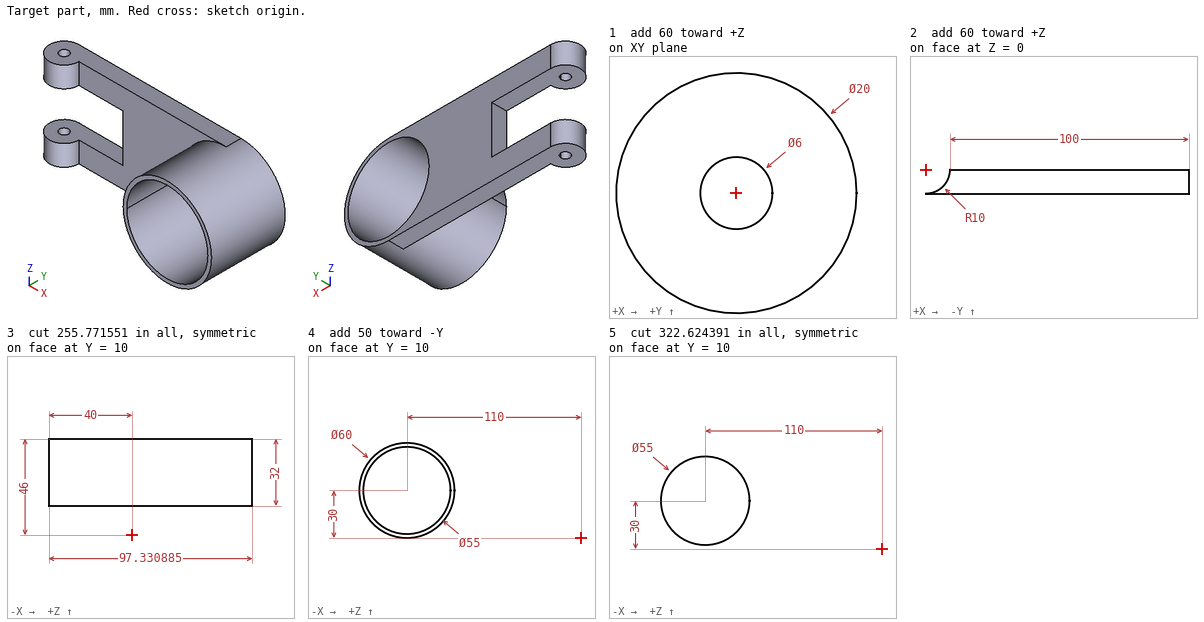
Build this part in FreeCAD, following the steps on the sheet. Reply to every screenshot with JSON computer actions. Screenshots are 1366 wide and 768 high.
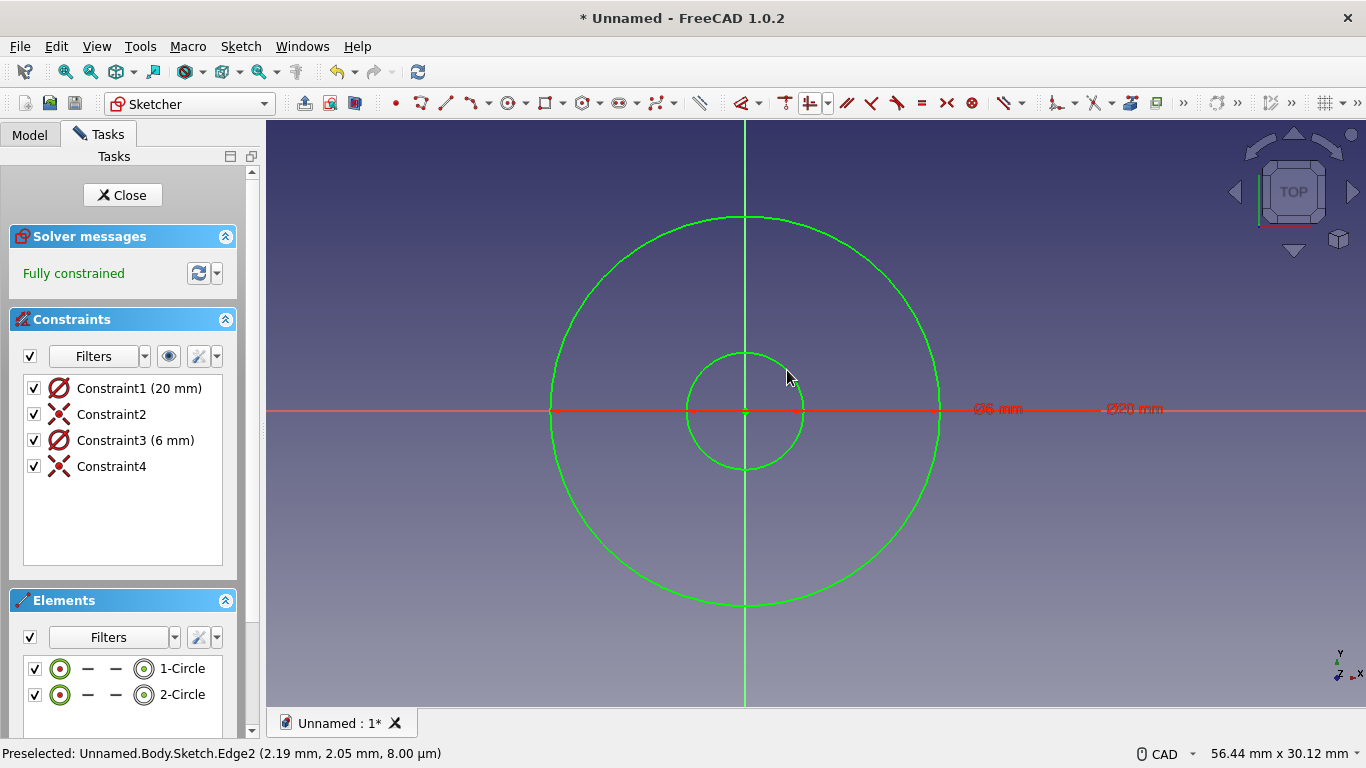
{"action": "left_click", "coordinate": [123, 195]}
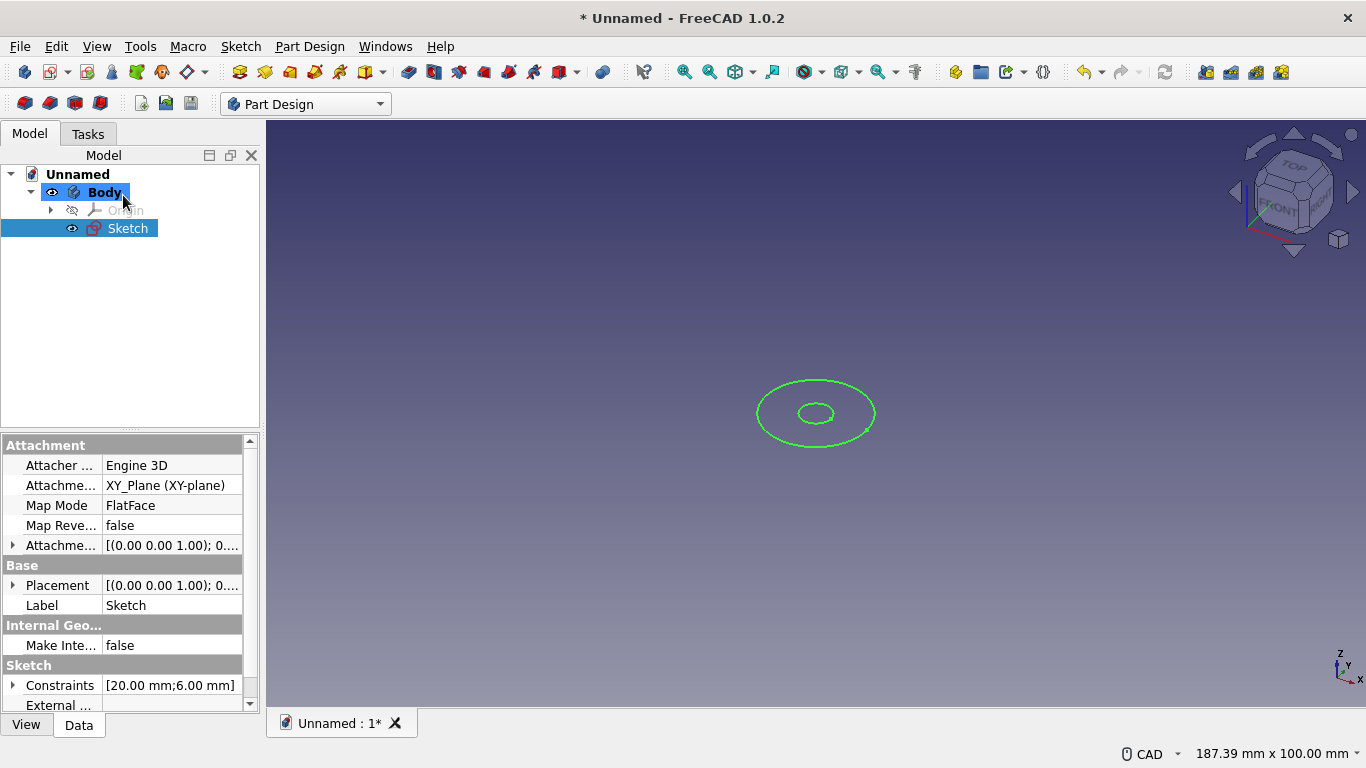
{"action": "left_click", "coordinate": [240, 72]}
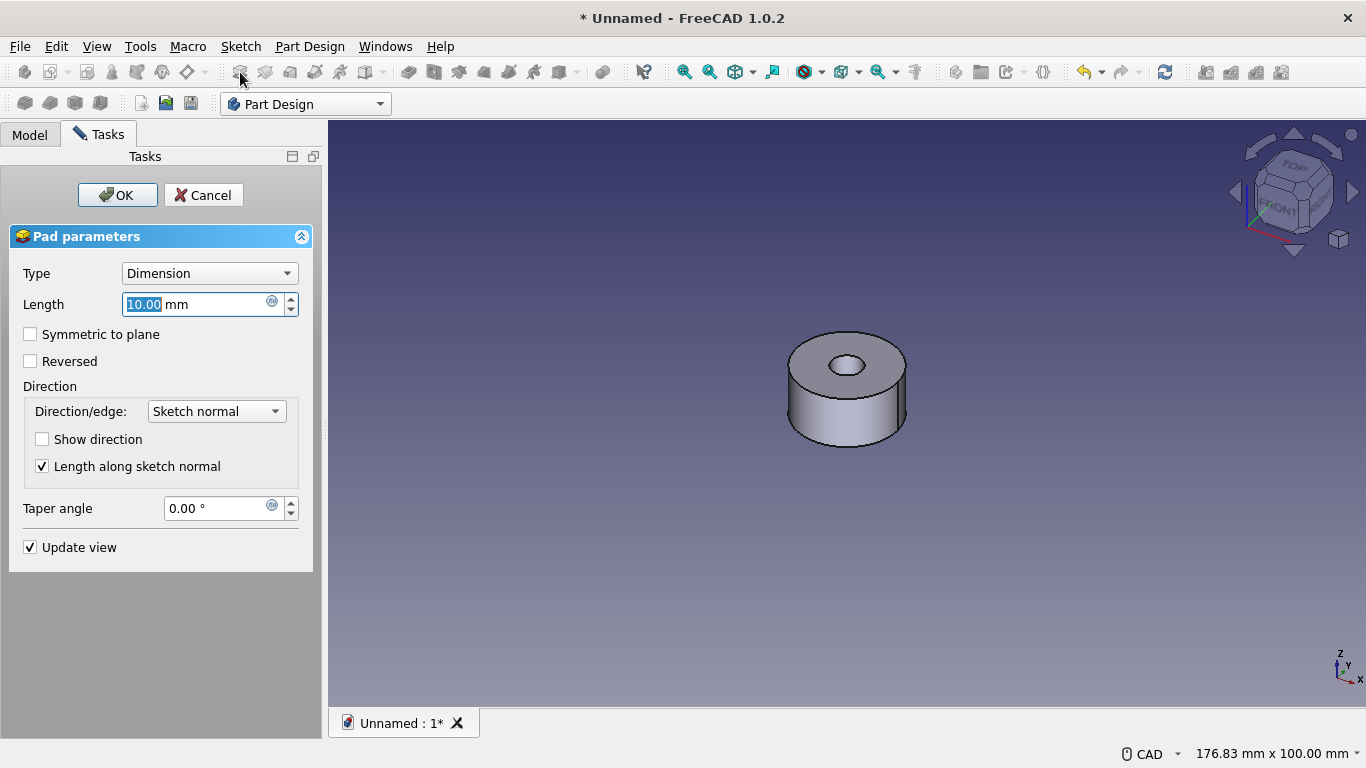
{"action": "type", "text": "60"}
{"action": "key", "text": "Tab"}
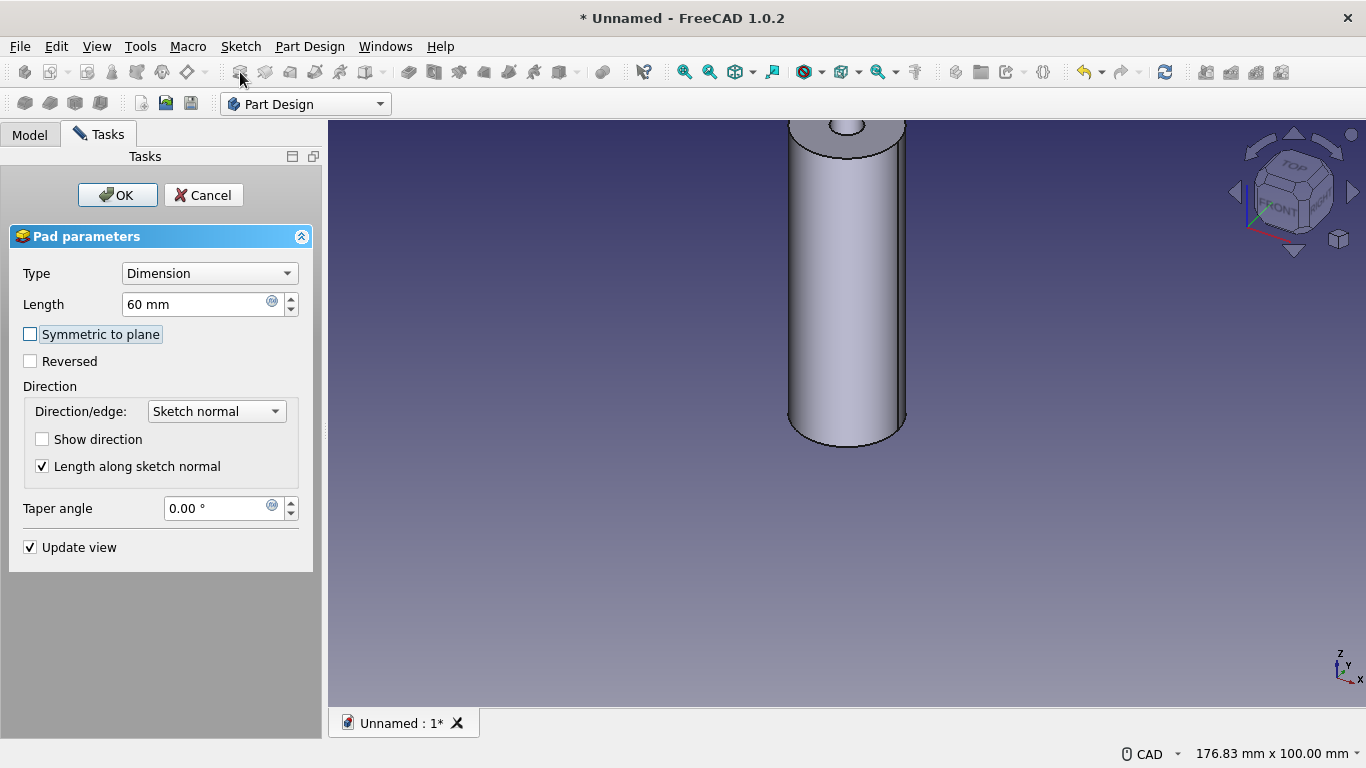
{"action": "left_click", "coordinate": [118, 195]}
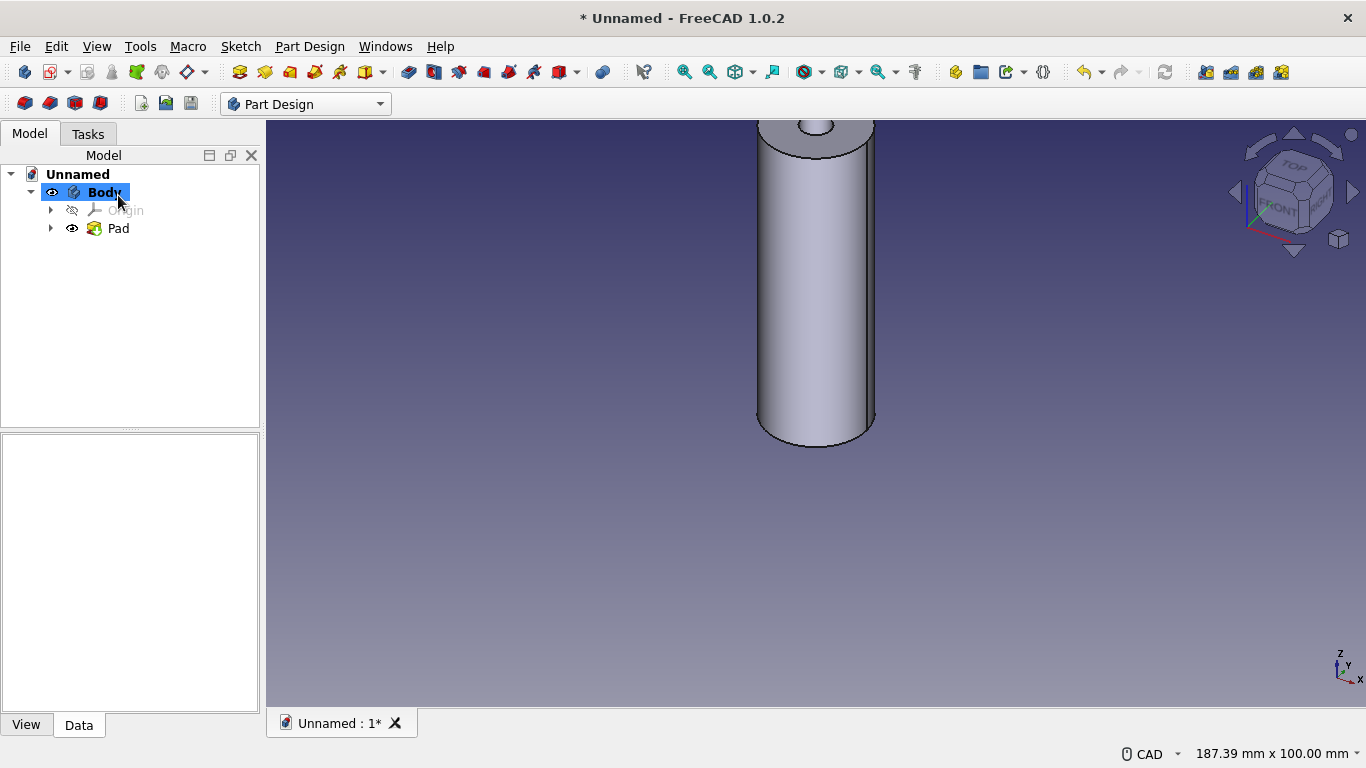
{"action": "left_click", "coordinate": [685, 72]}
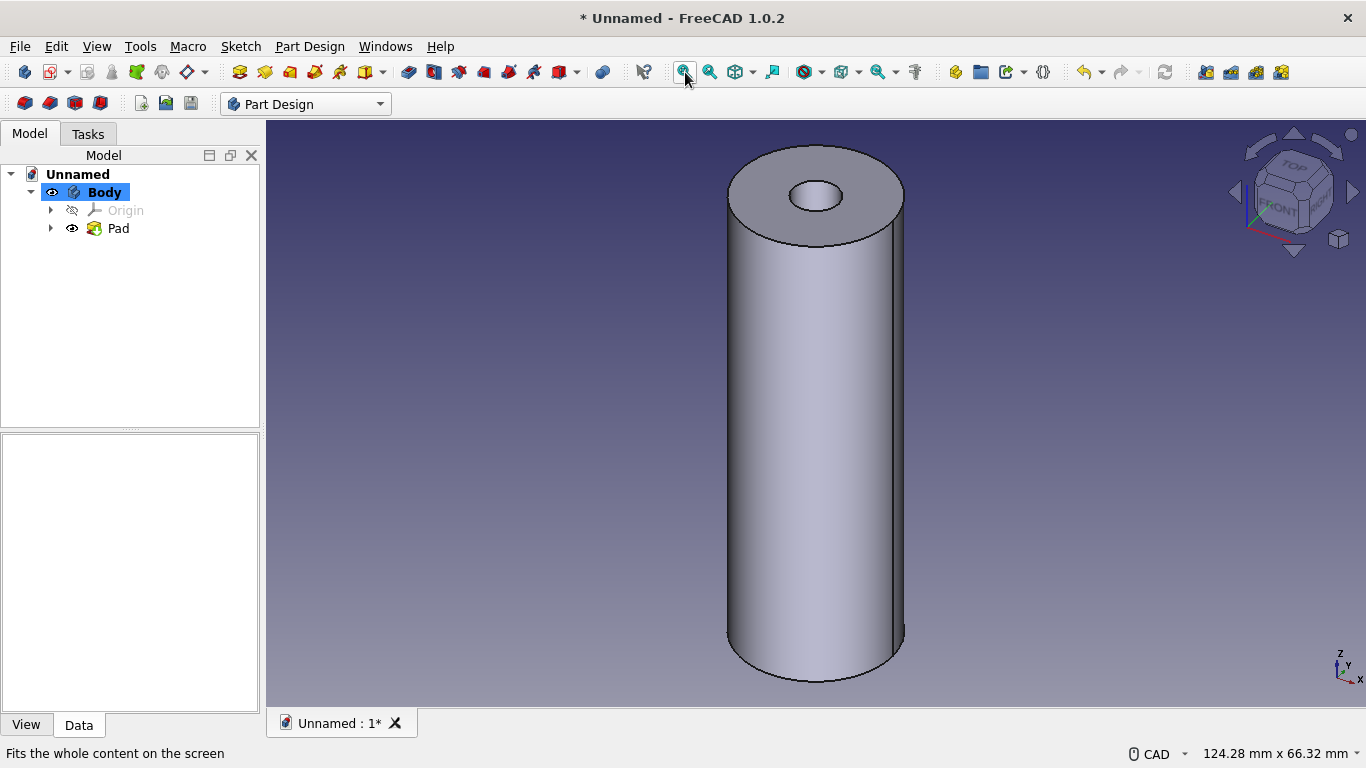
{"action": "key", "text": "5"}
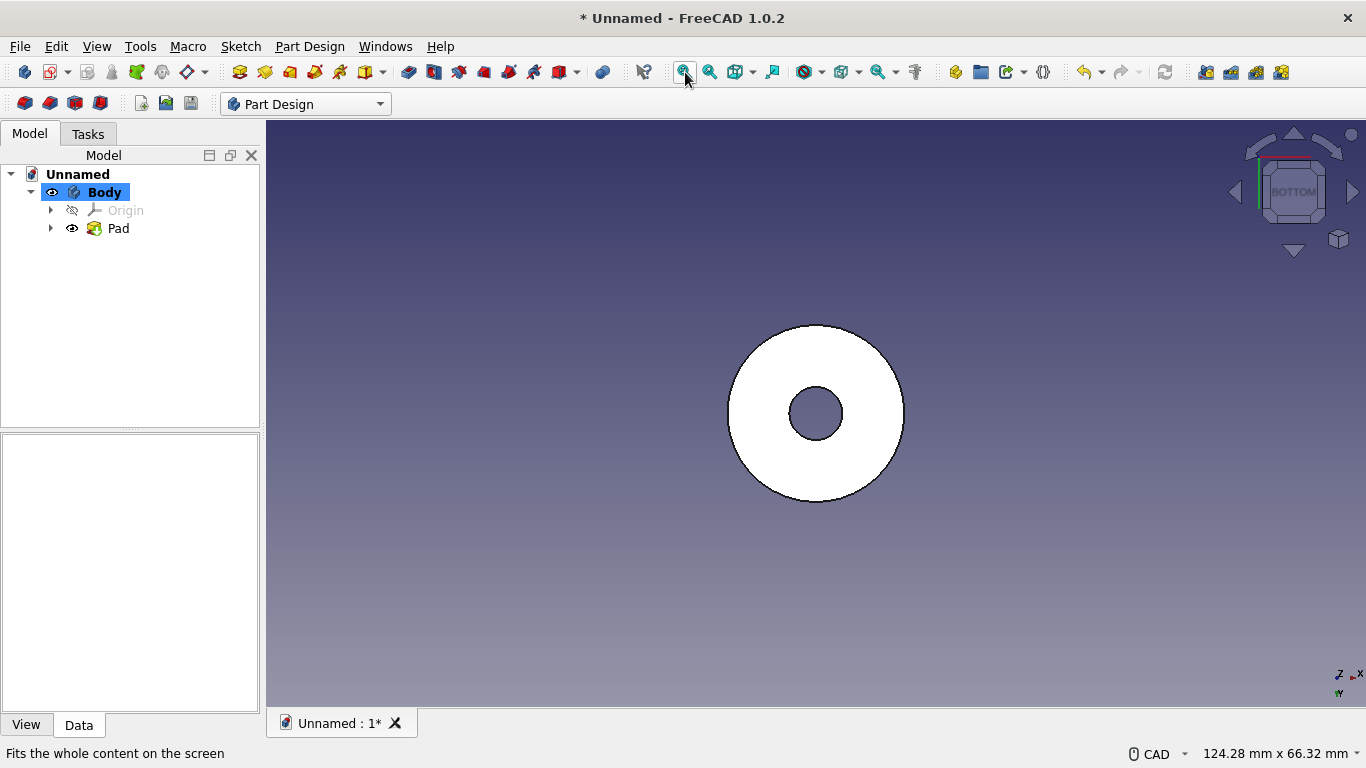
{"action": "left_click", "coordinate": [685, 72]}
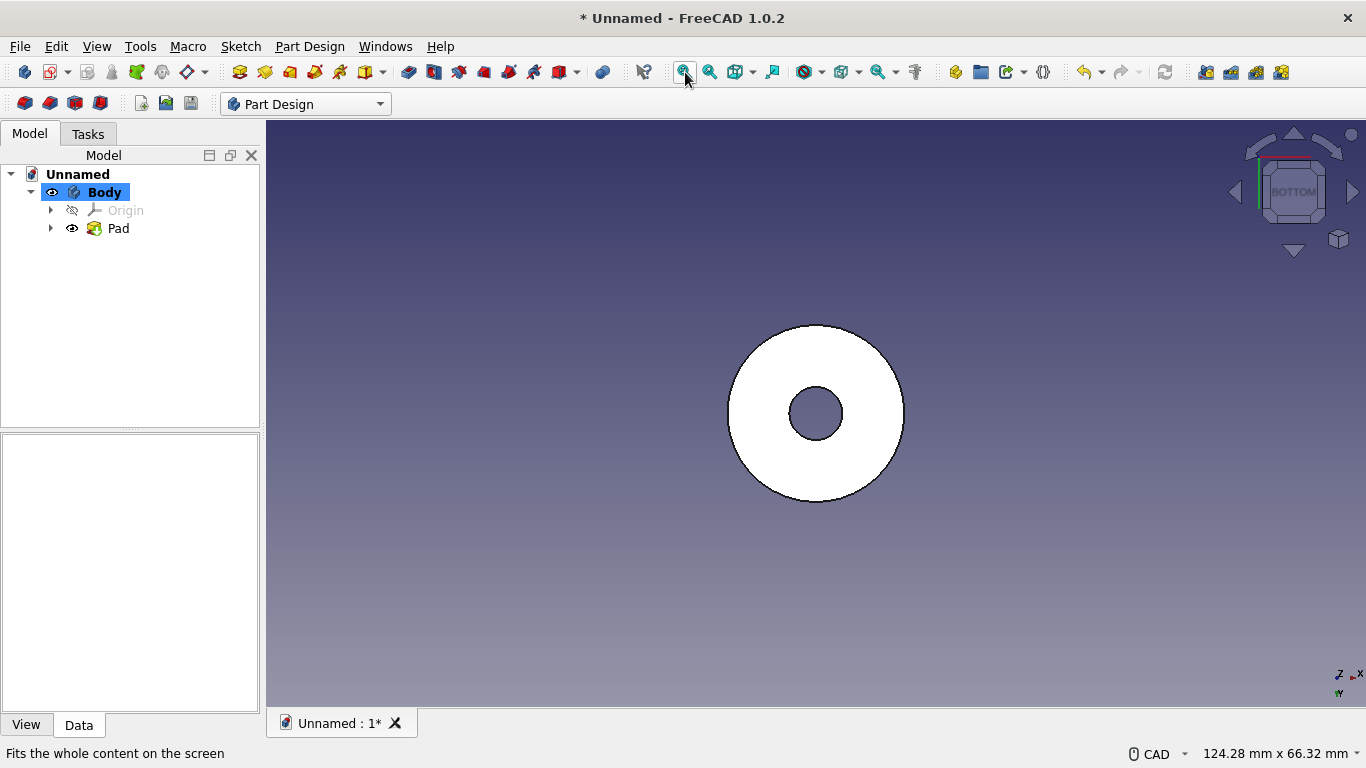
{"action": "left_click", "coordinate": [765, 438]}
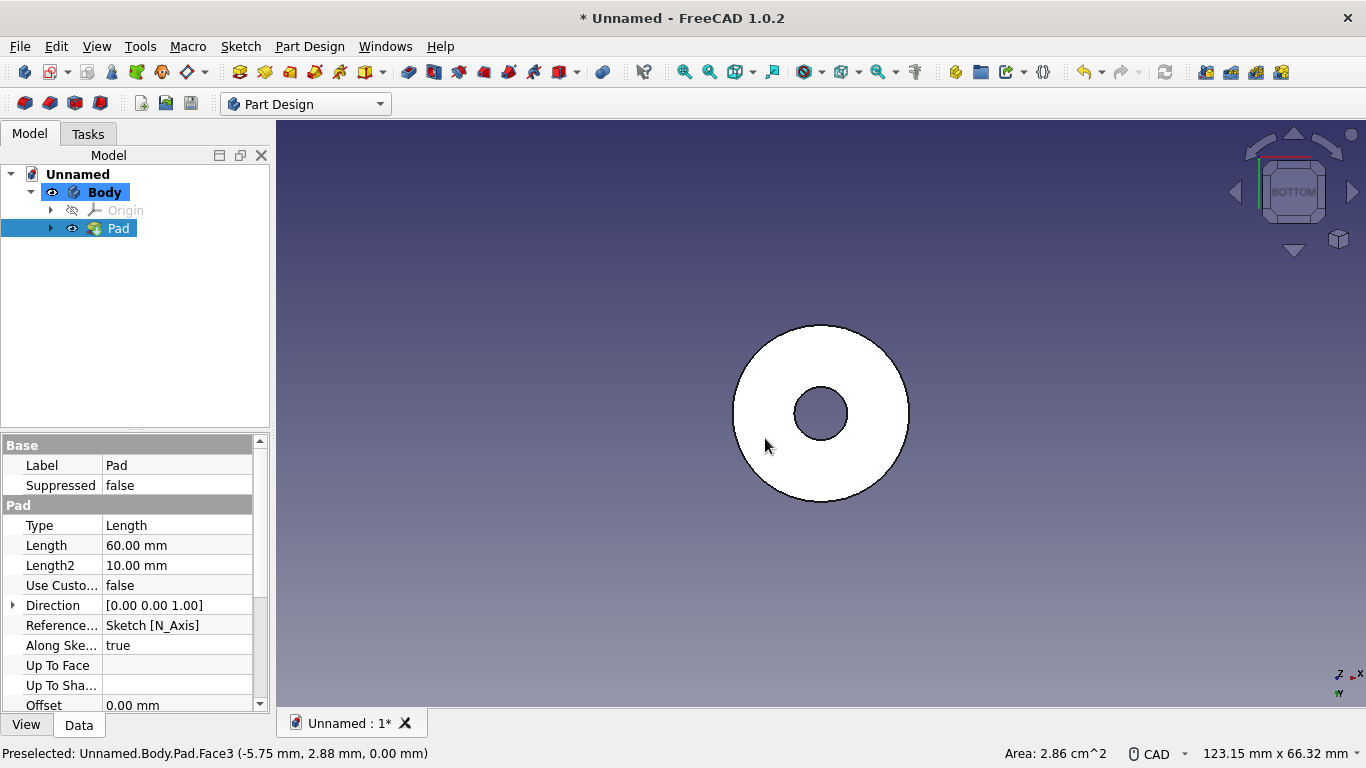
{"action": "left_click", "coordinate": [50, 72]}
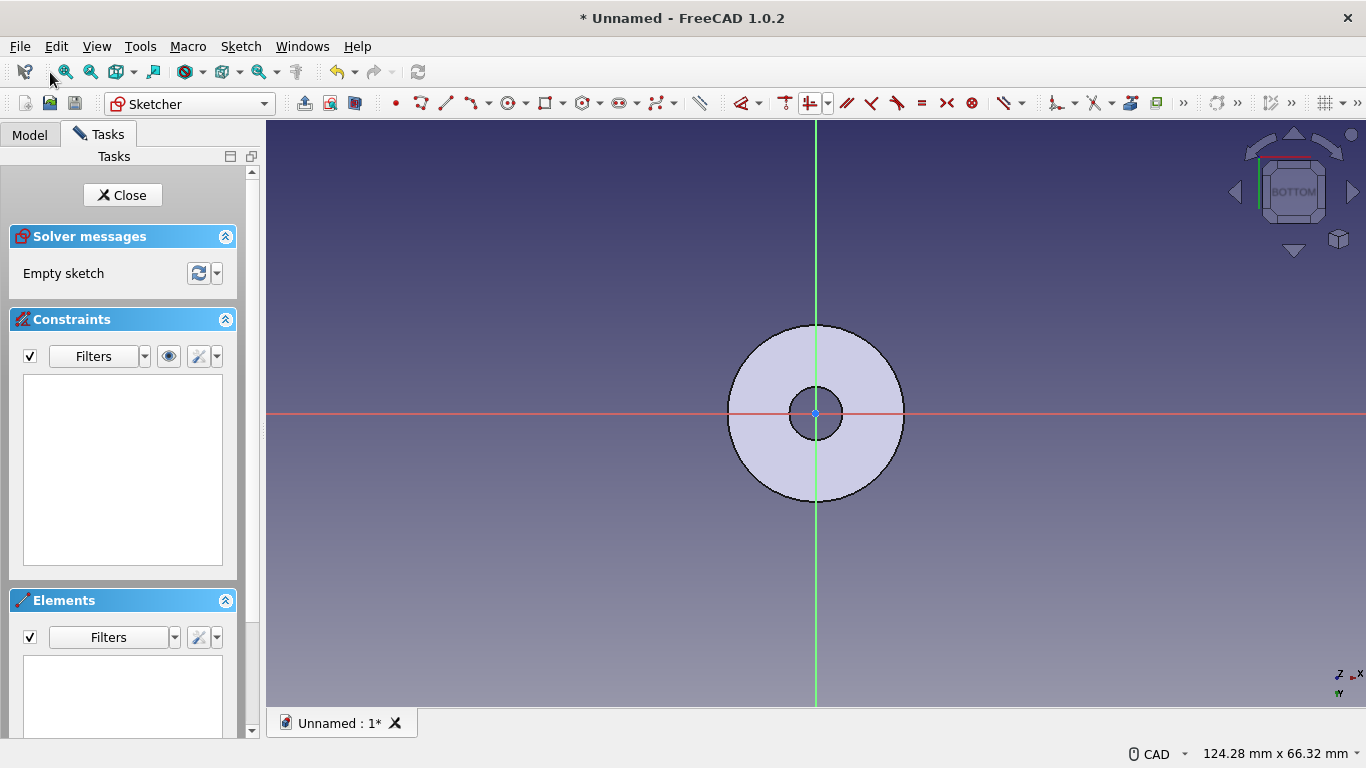
{"action": "scroll", "coordinate": [294, 360], "scroll_direction": "down", "scroll_amount": 3}